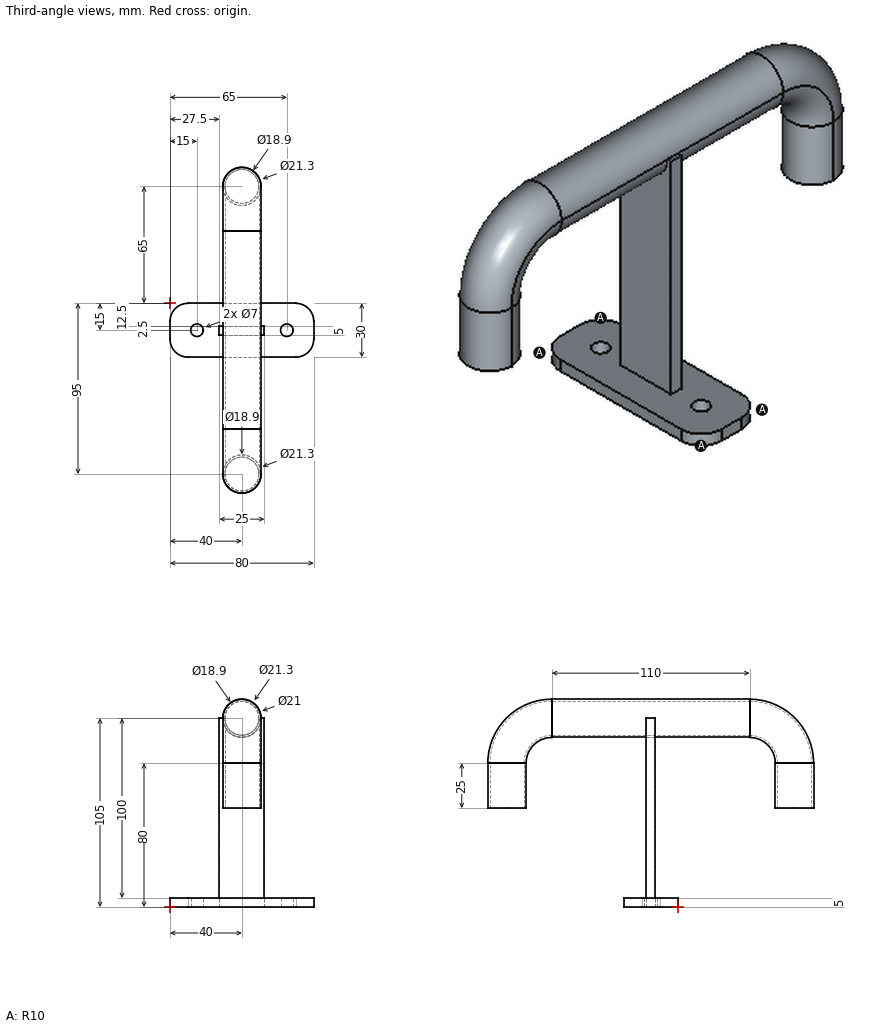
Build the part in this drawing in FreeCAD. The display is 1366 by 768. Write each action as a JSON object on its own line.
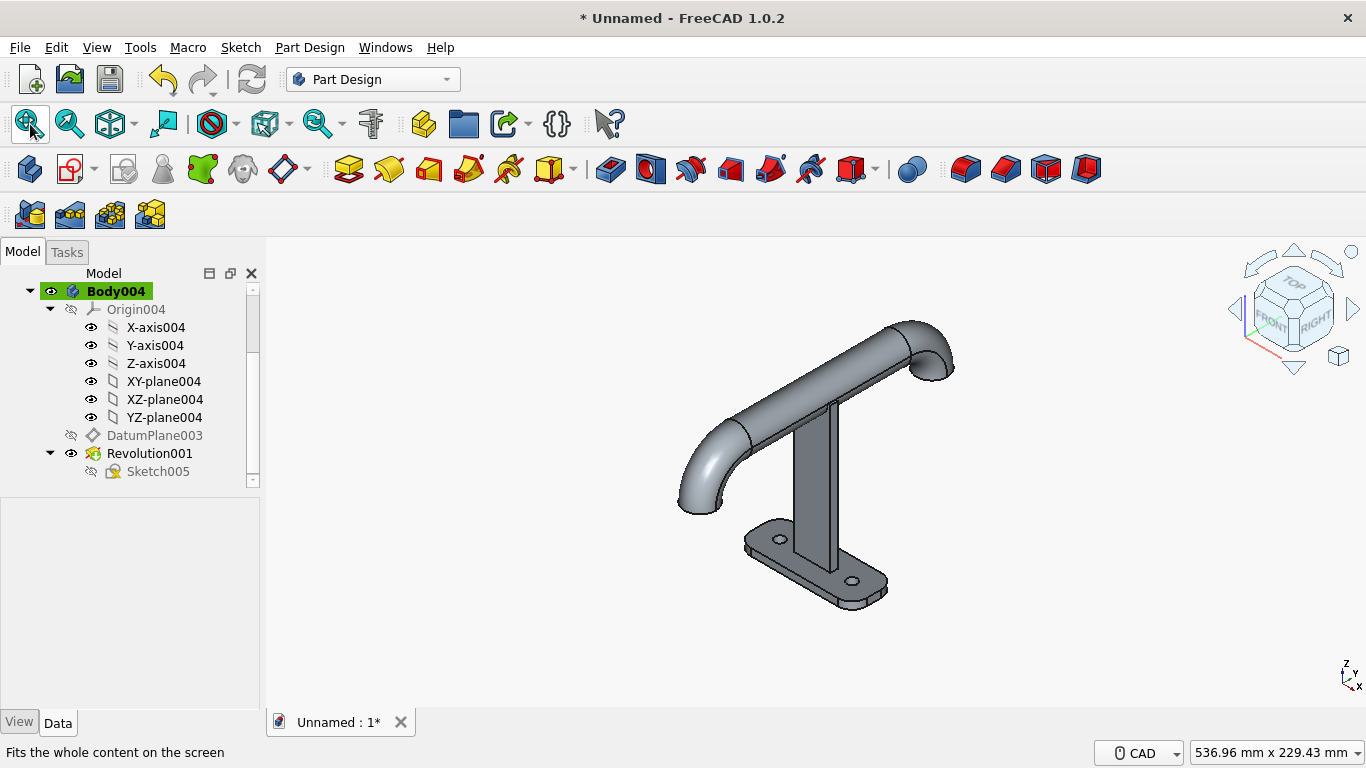
{"action": "left_click", "coordinate": [30, 170]}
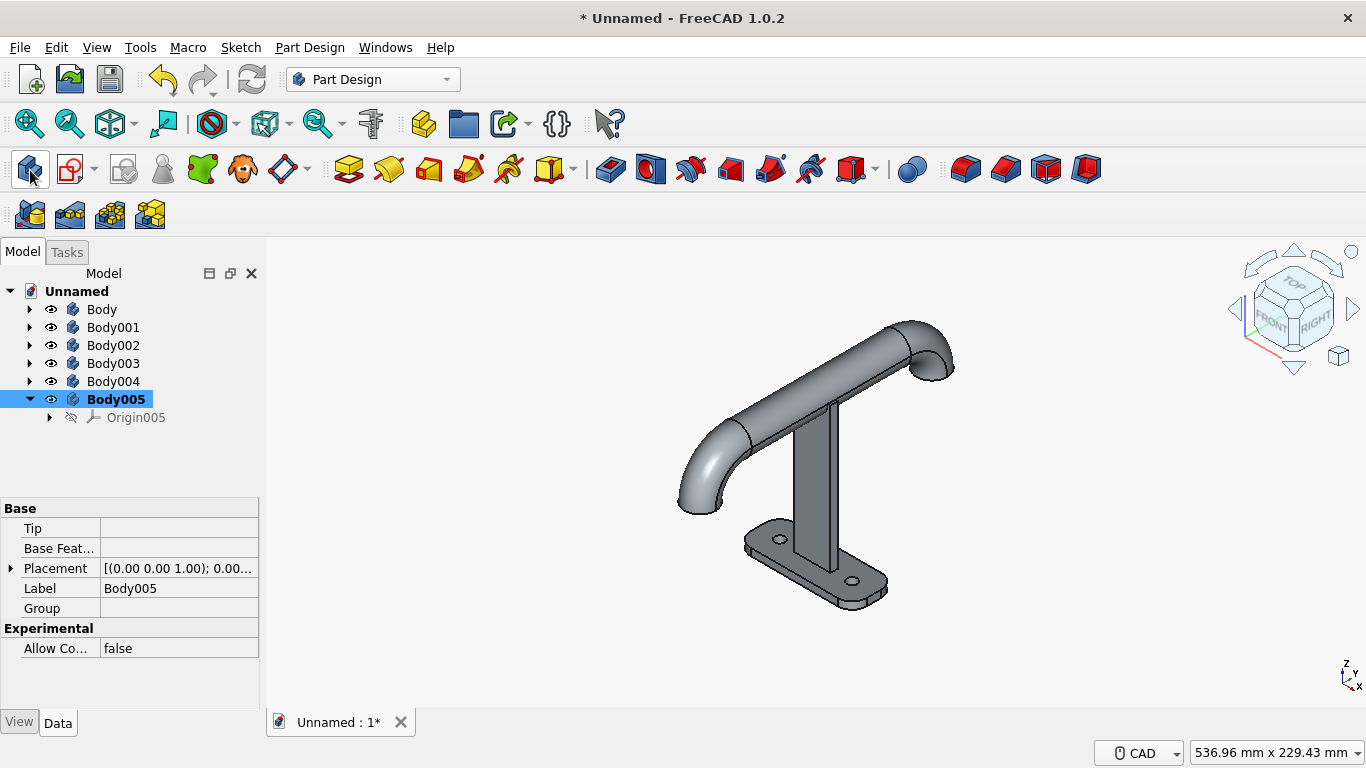
{"action": "left_click", "coordinate": [50, 417]}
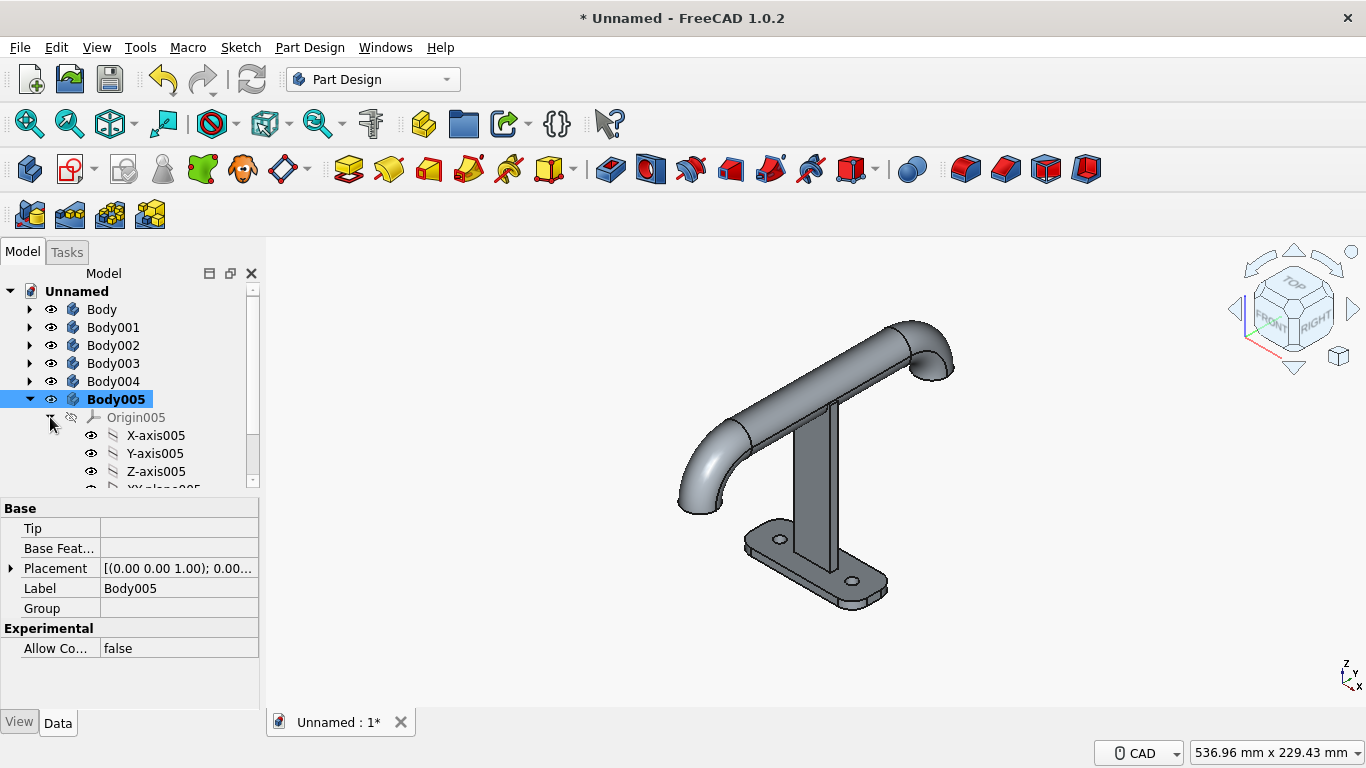
{"action": "scroll", "coordinate": [100, 377], "scroll_direction": "down", "scroll_amount": 3}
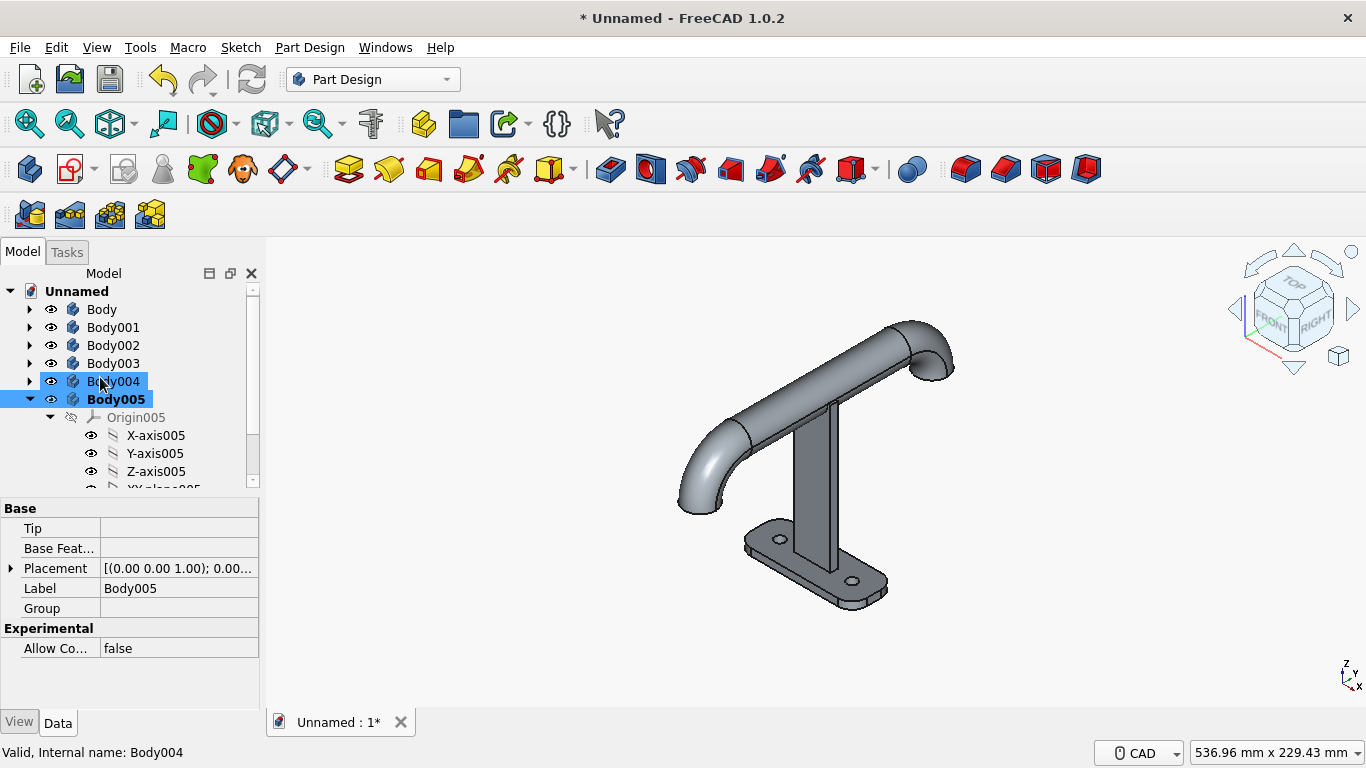
{"action": "left_click", "coordinate": [136, 435]}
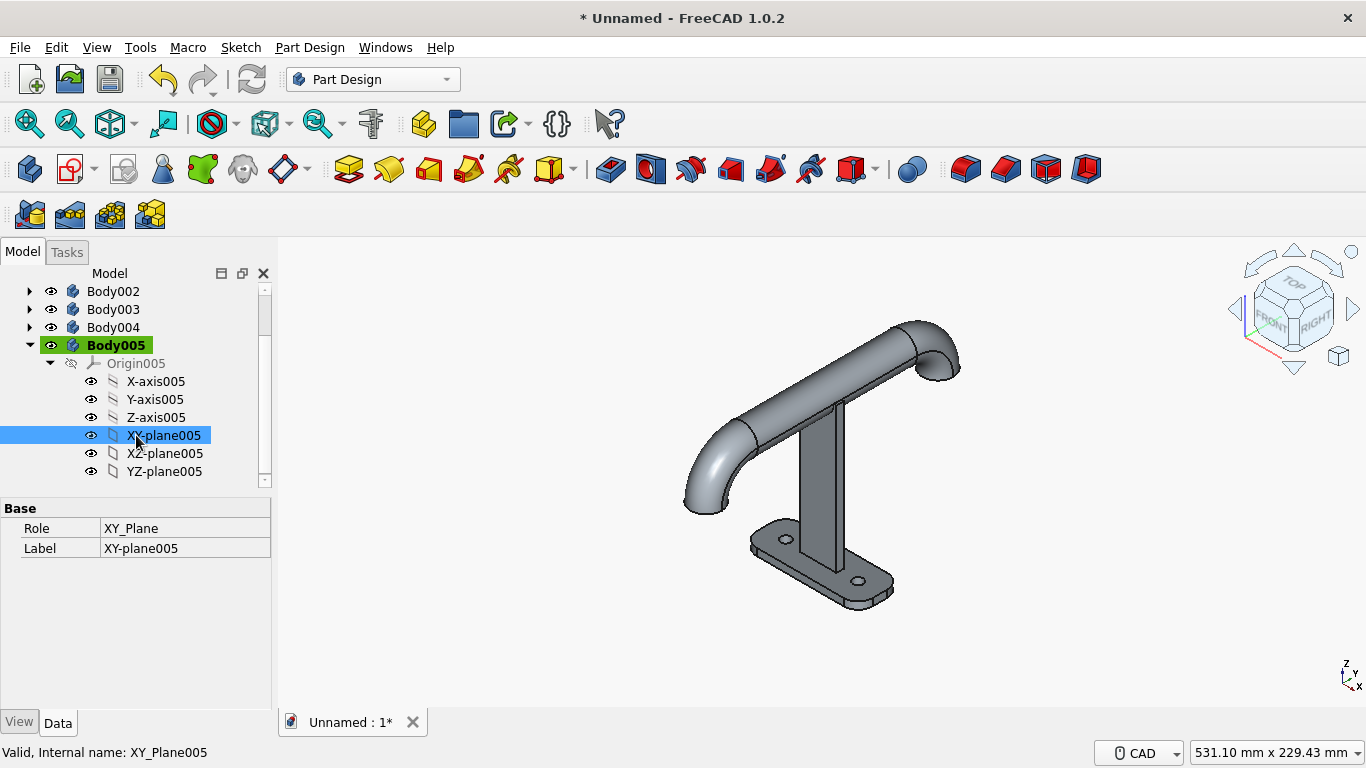
{"action": "left_click", "coordinate": [284, 170]}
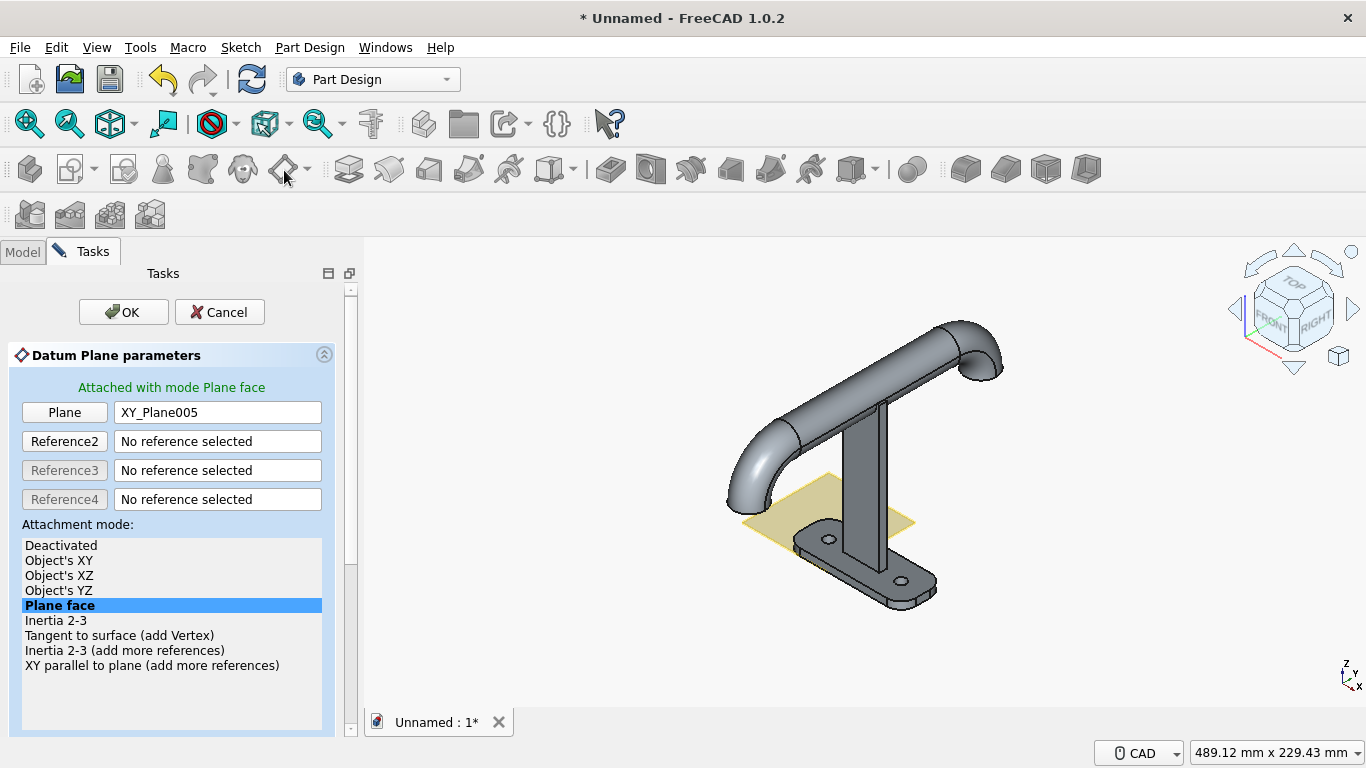
{"action": "scroll", "coordinate": [351, 510], "scroll_direction": "down", "scroll_amount": 3}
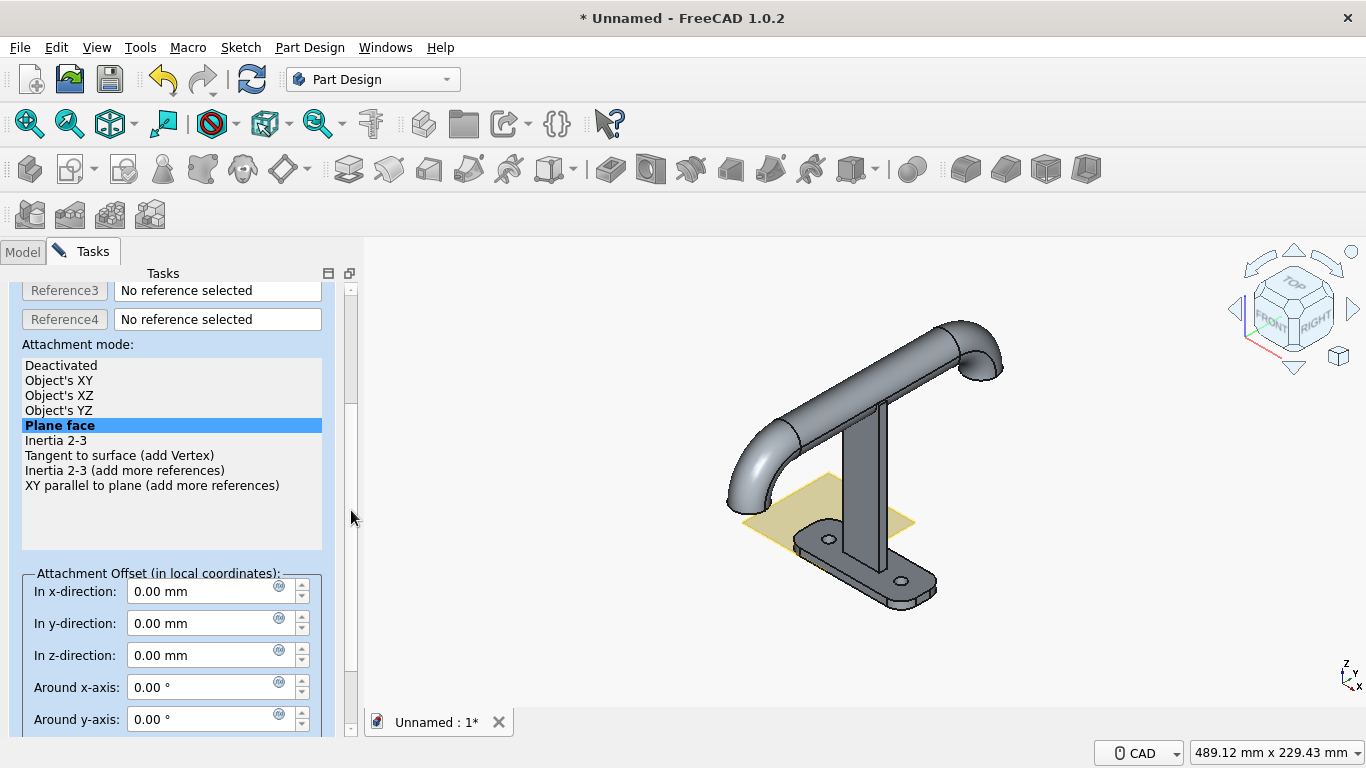
{"action": "triple_click", "coordinate": [210, 655]}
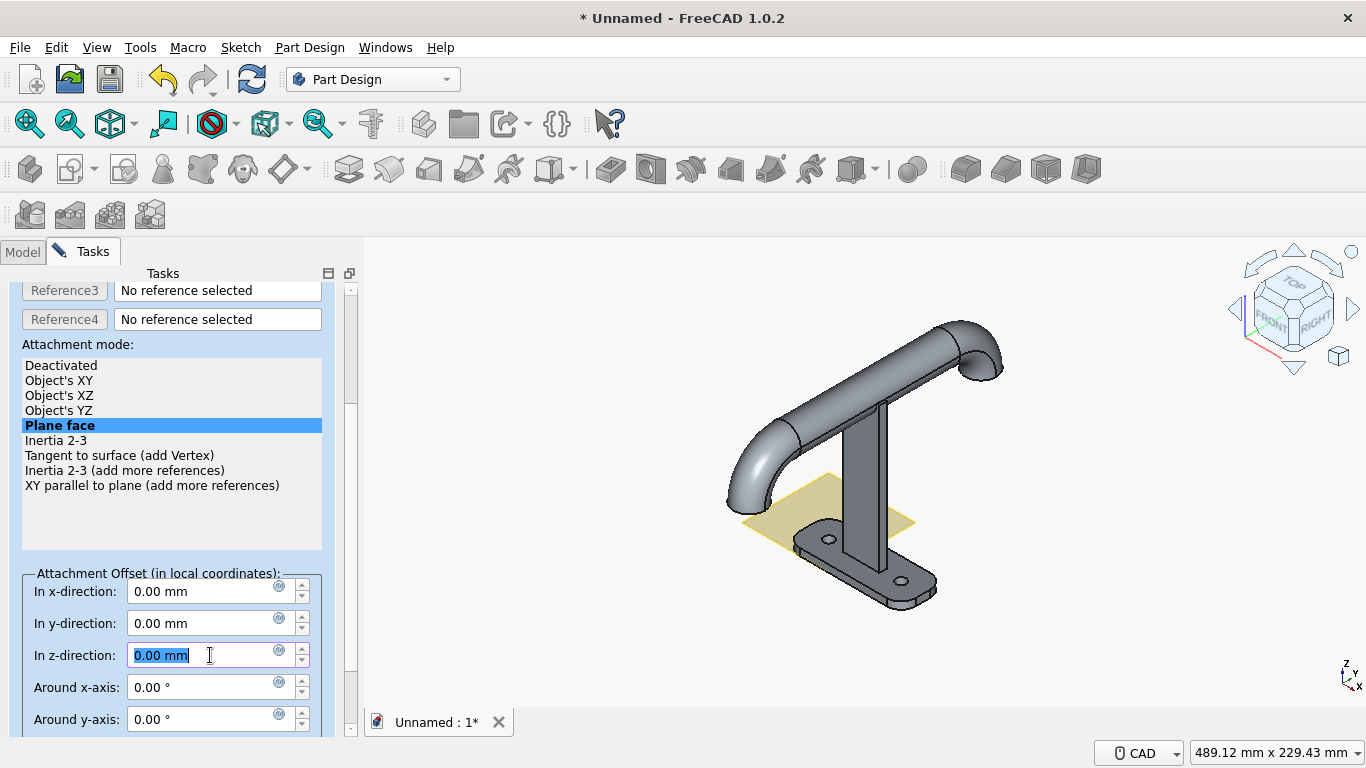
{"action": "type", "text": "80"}
{"action": "key", "text": "Tab"}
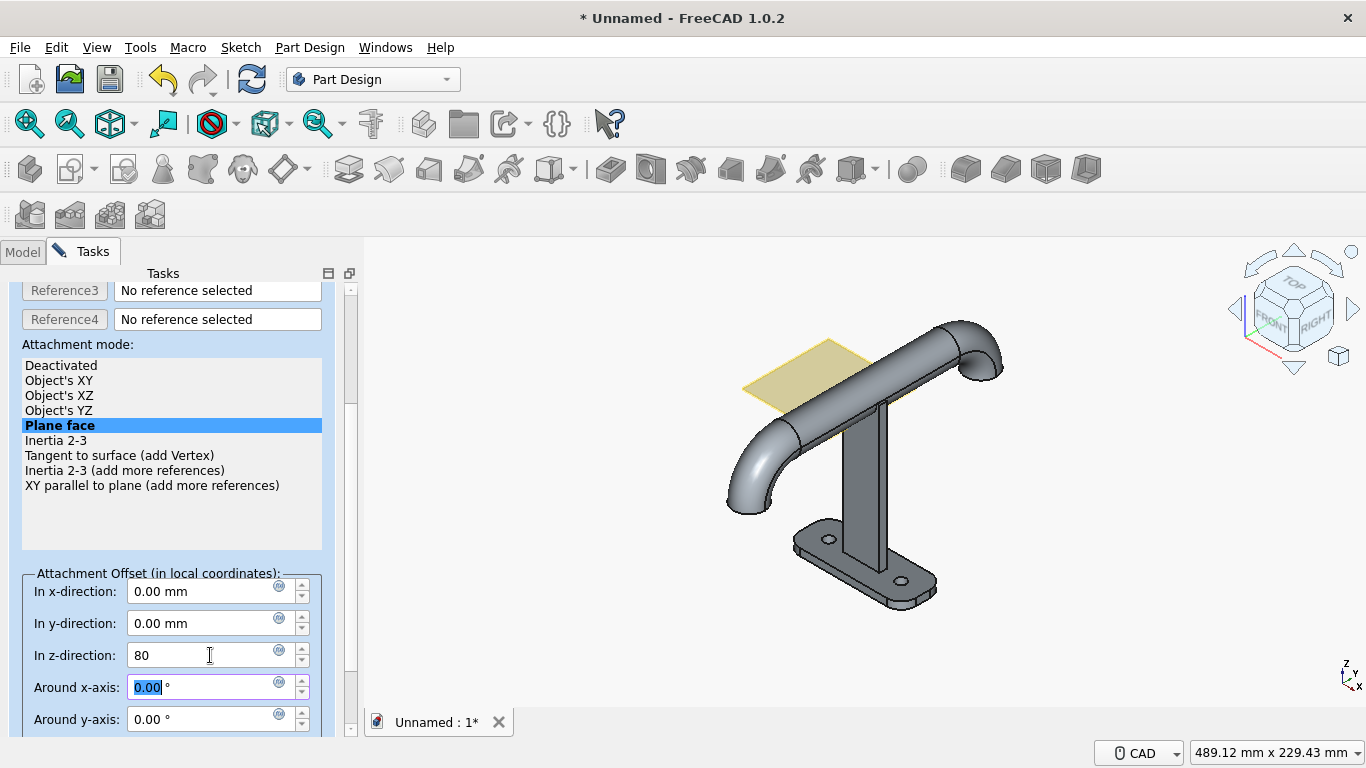
{"action": "scroll", "coordinate": [351, 510], "scroll_direction": "up", "scroll_amount": 4}